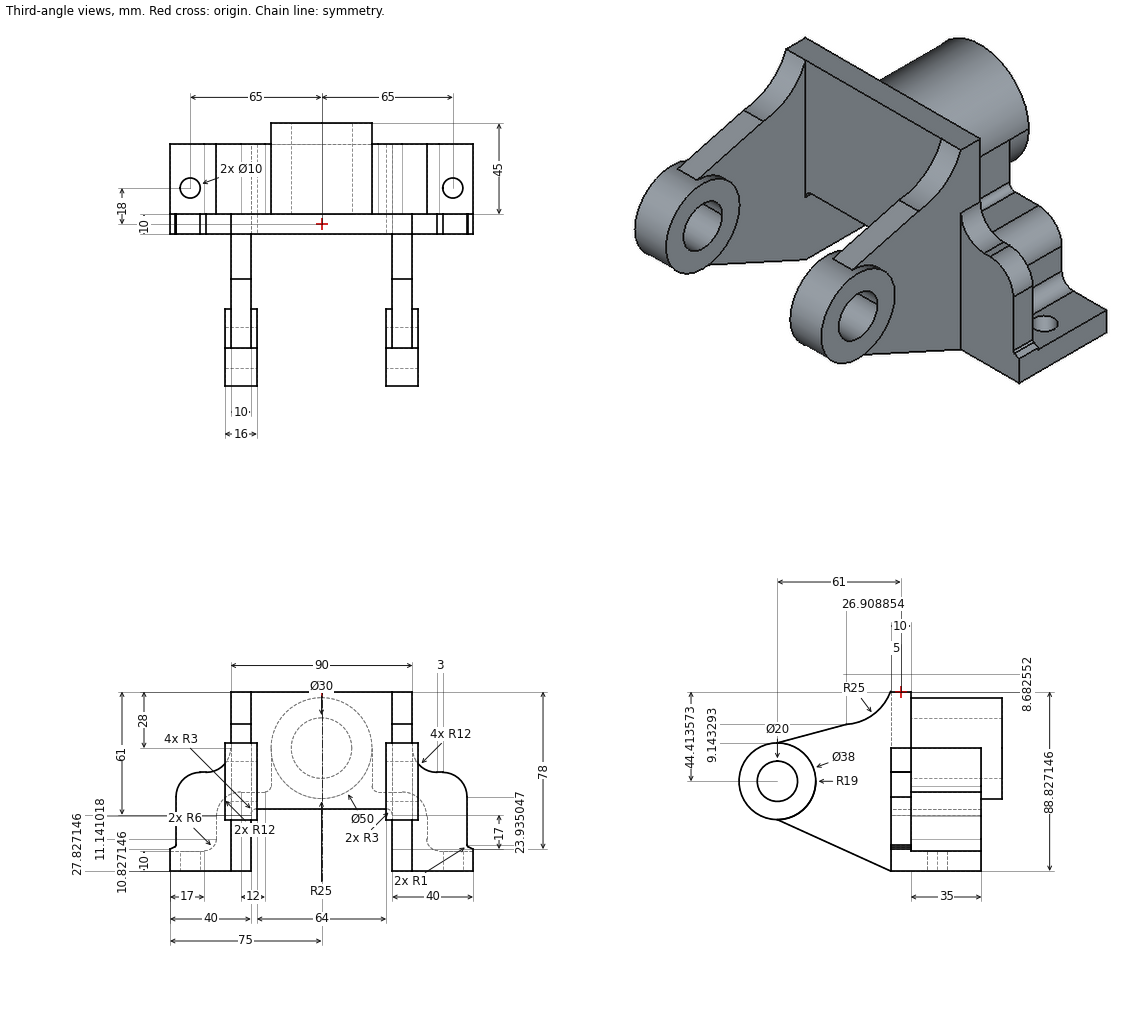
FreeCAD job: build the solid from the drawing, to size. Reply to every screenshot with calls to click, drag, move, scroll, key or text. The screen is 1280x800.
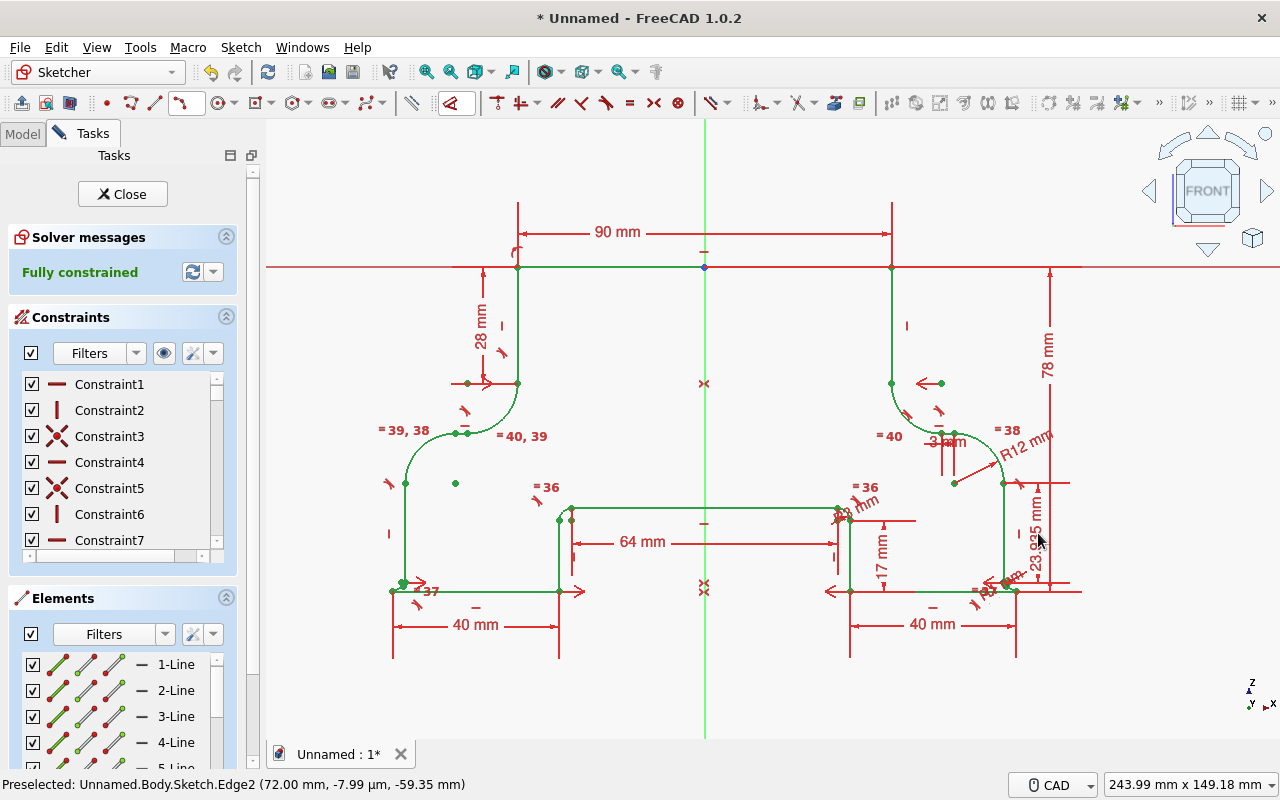
click(123, 194)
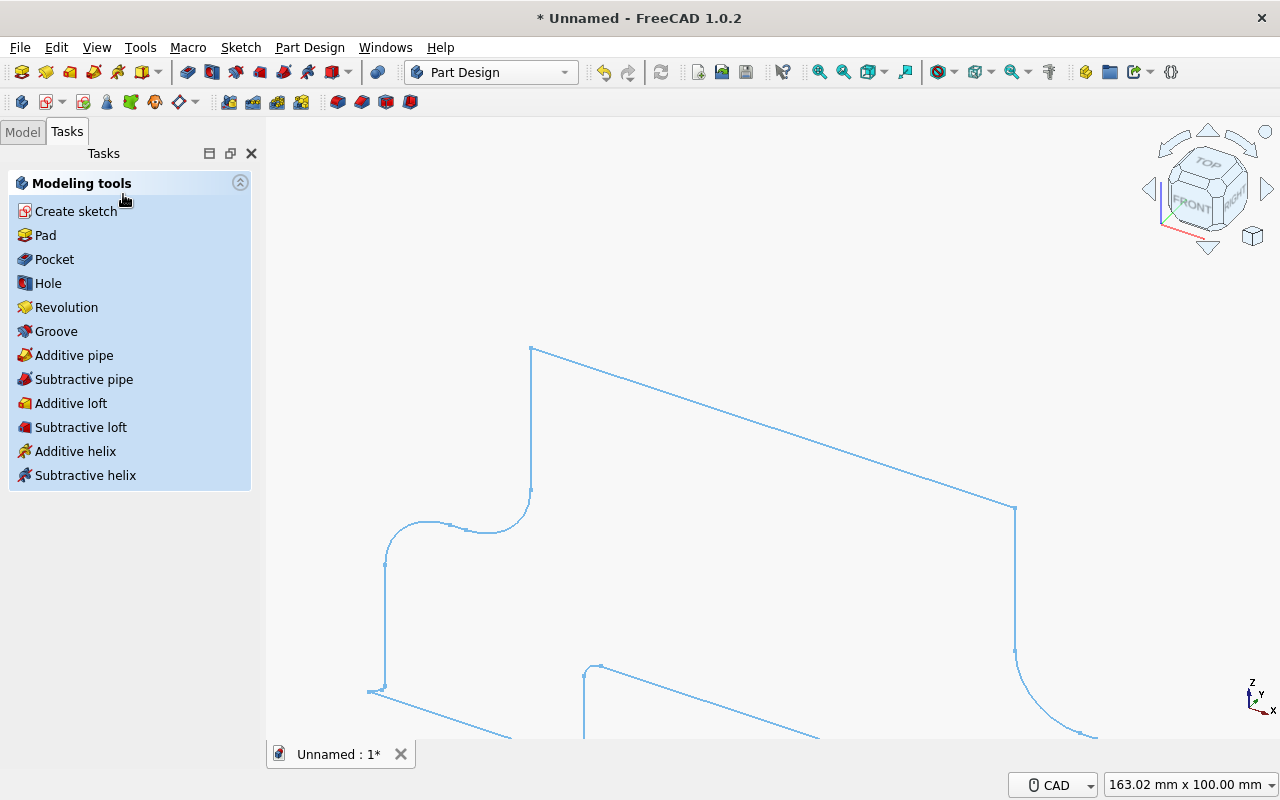
click(22, 72)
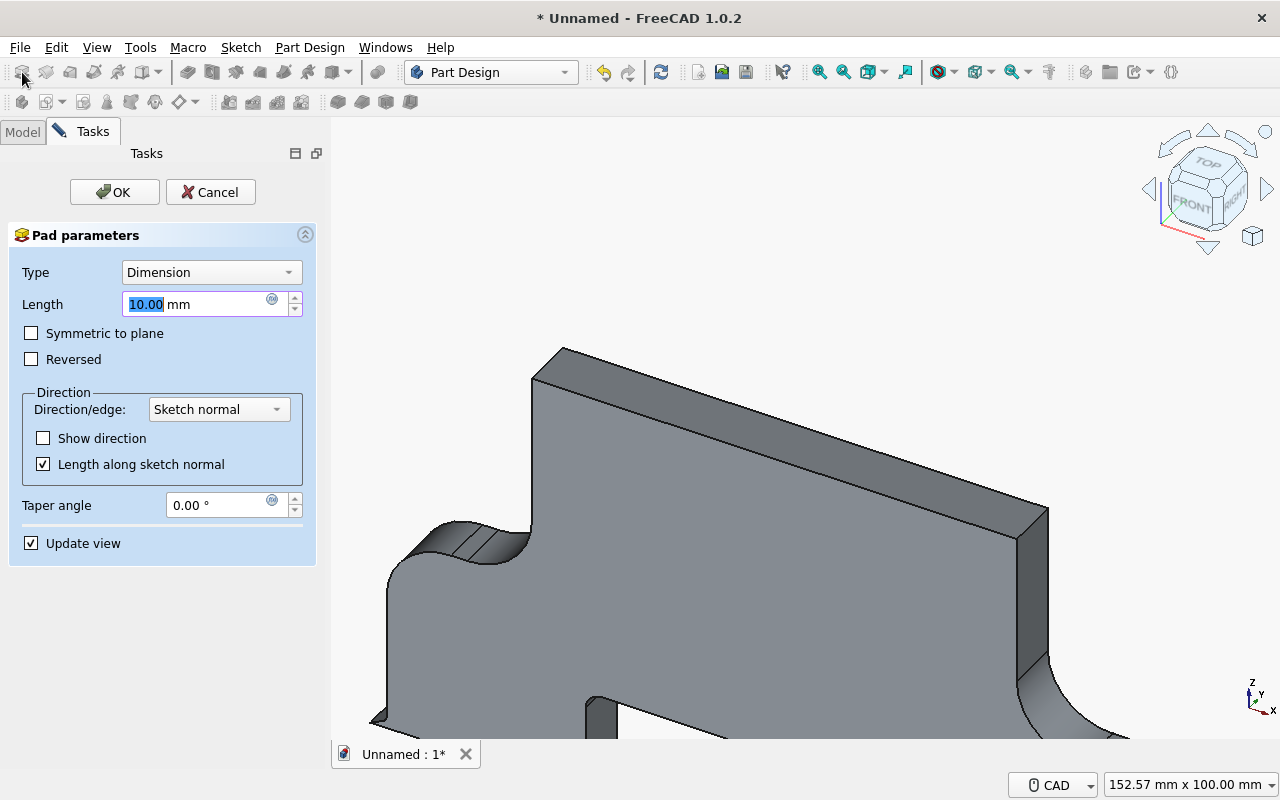
text(10)
key(Tab)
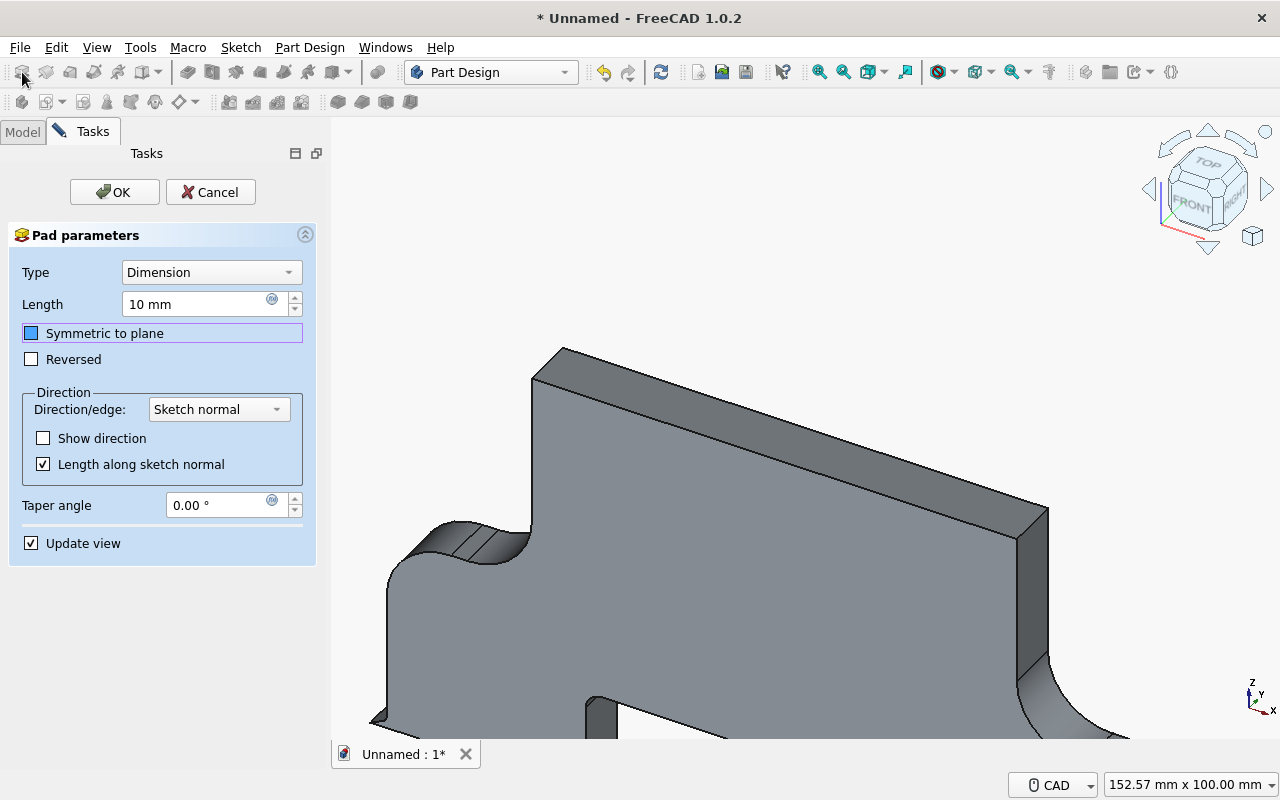
click(30, 333)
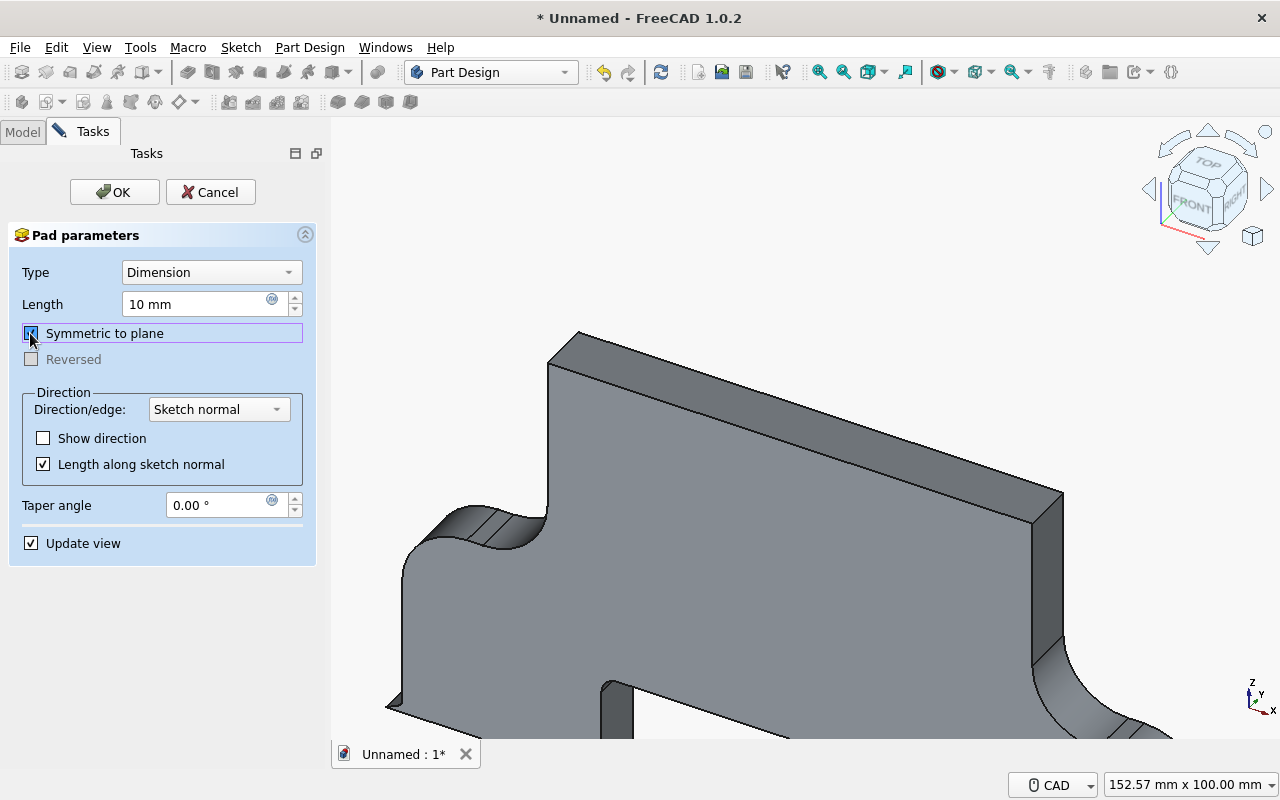
click(115, 192)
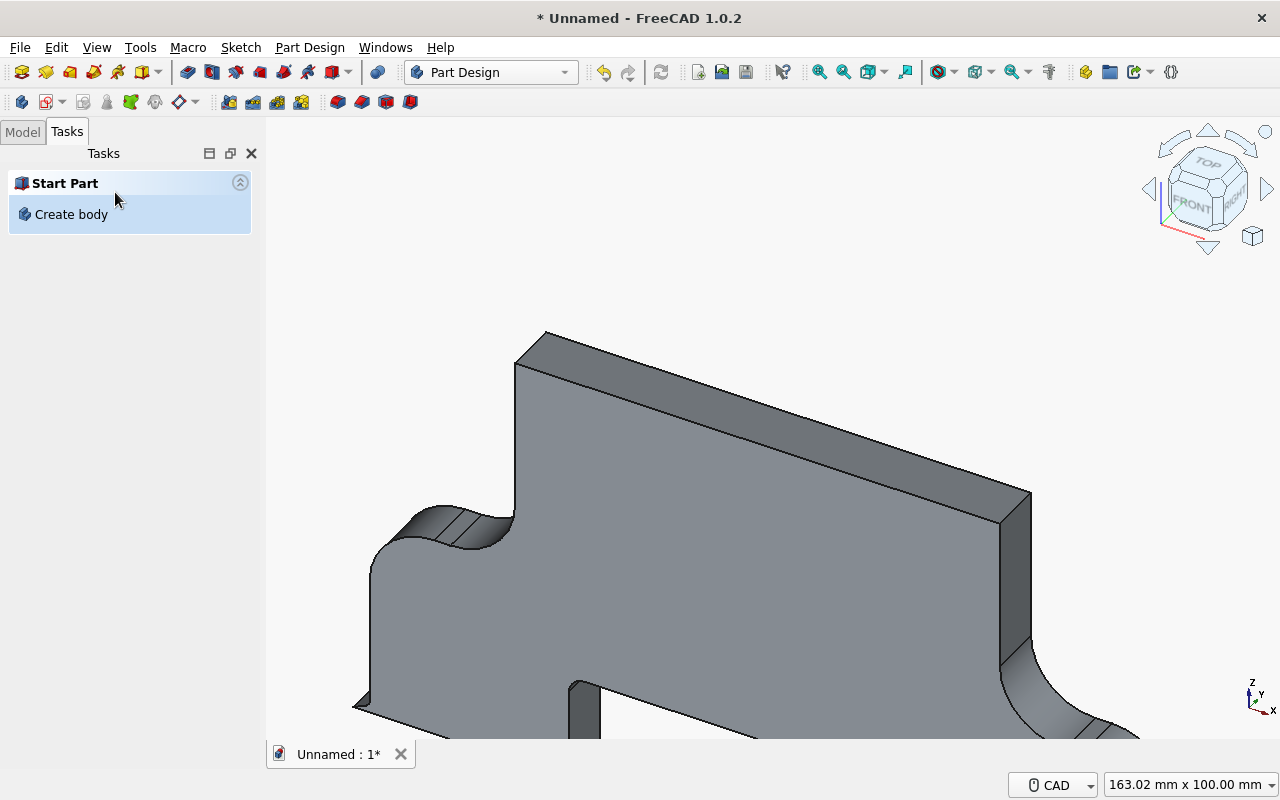
key(v)
key(f)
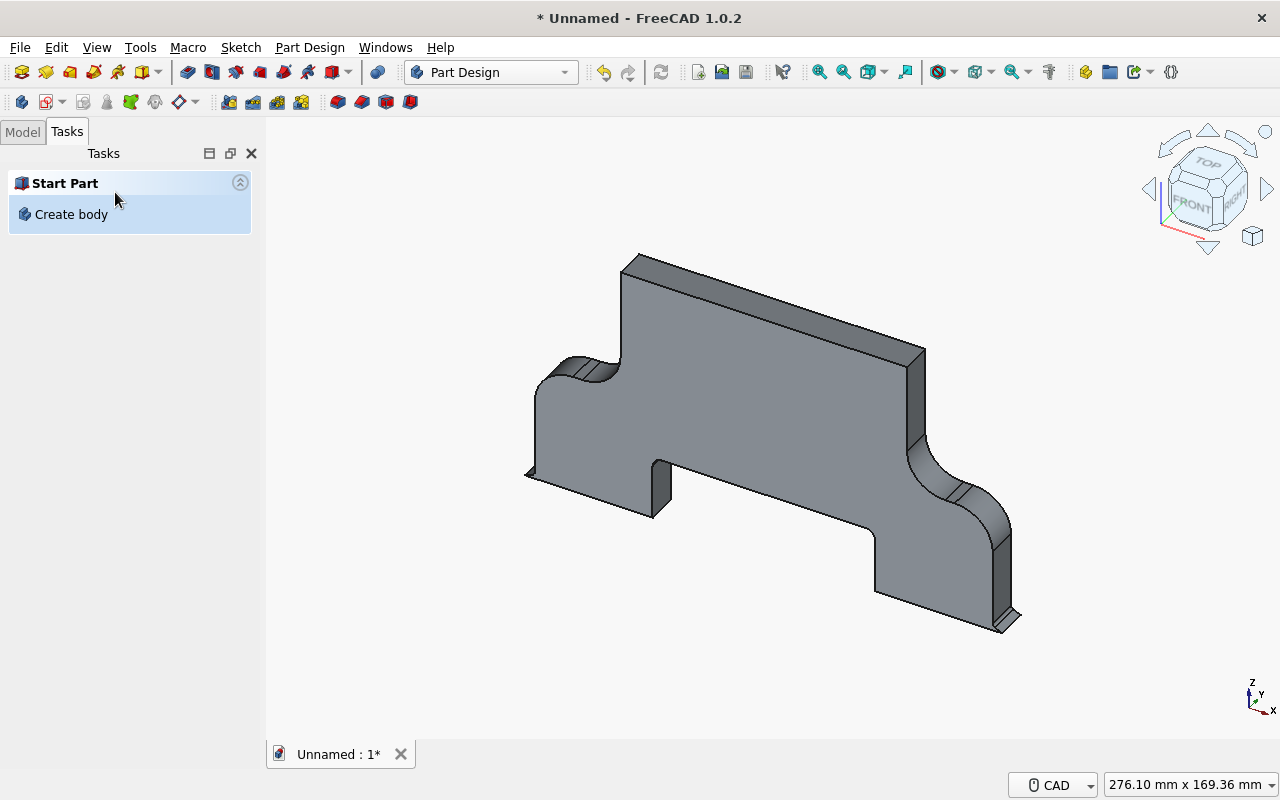
key(4)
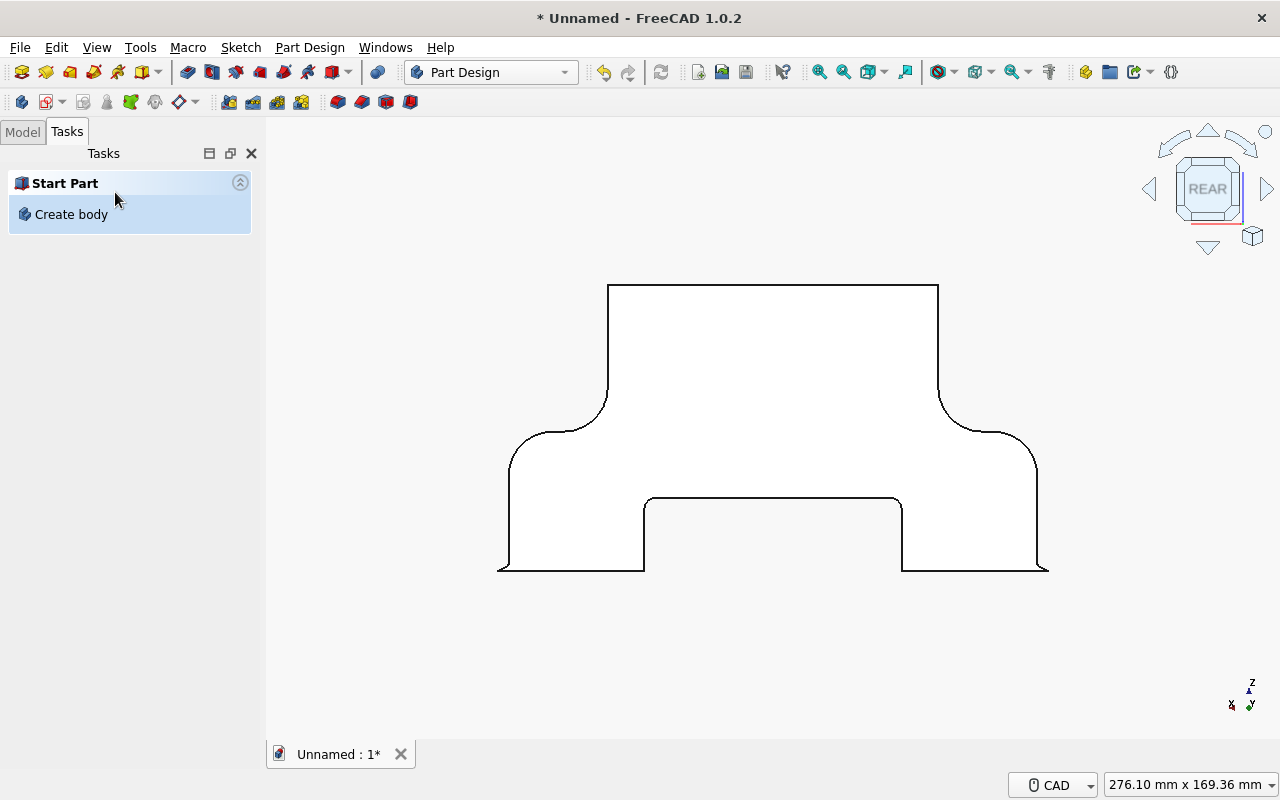
click(773, 386)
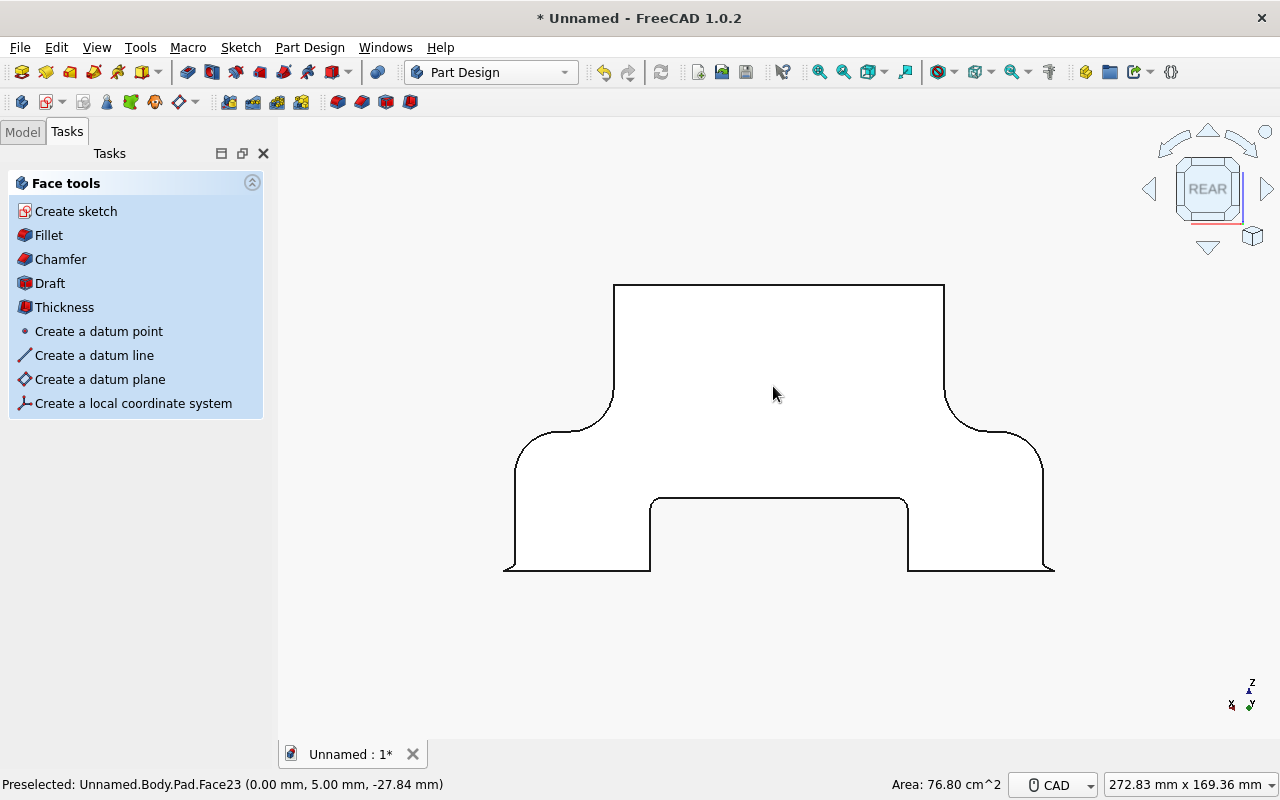
click(46, 102)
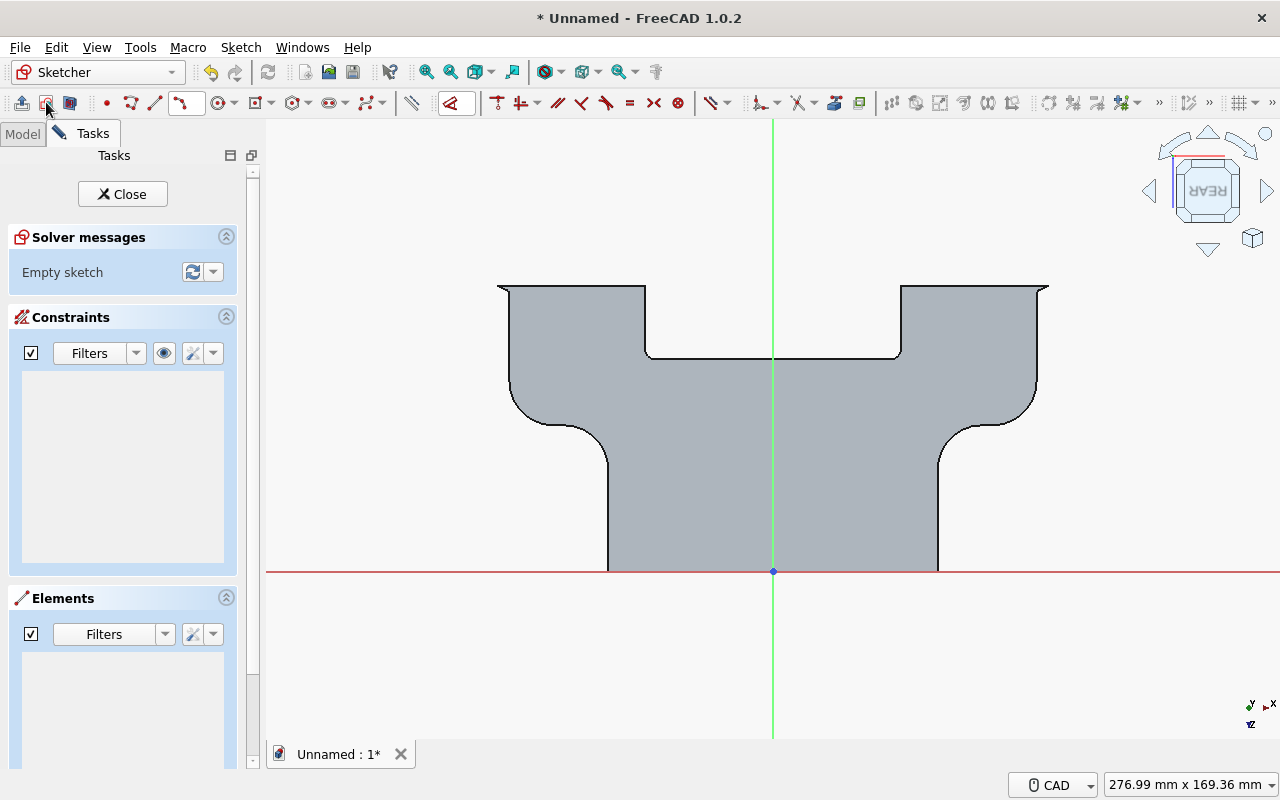
key(g)
key(r)